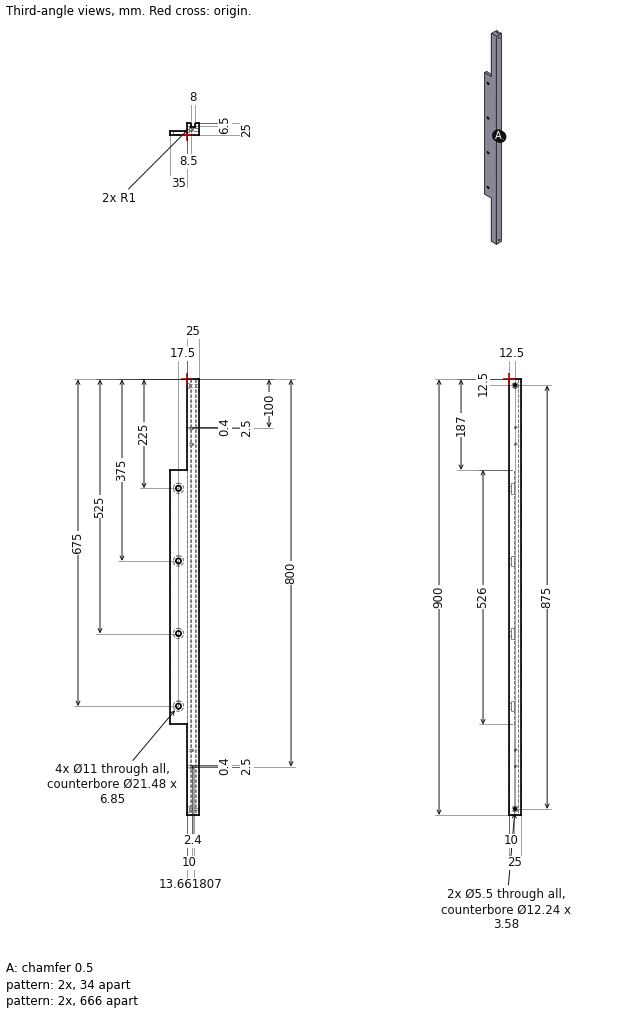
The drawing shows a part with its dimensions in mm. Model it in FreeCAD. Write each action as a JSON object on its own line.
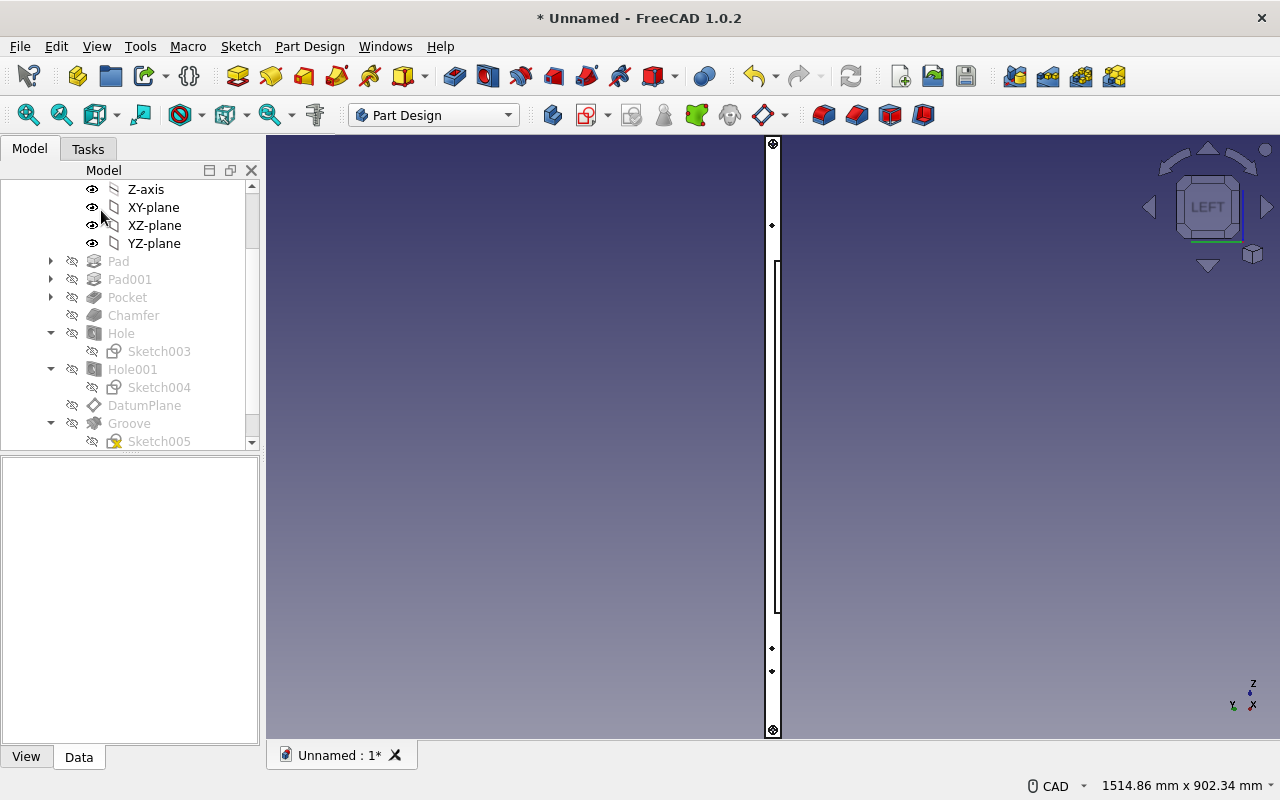
{"action": "scroll", "coordinate": [161, 311], "scroll_direction": "down", "scroll_amount": 3}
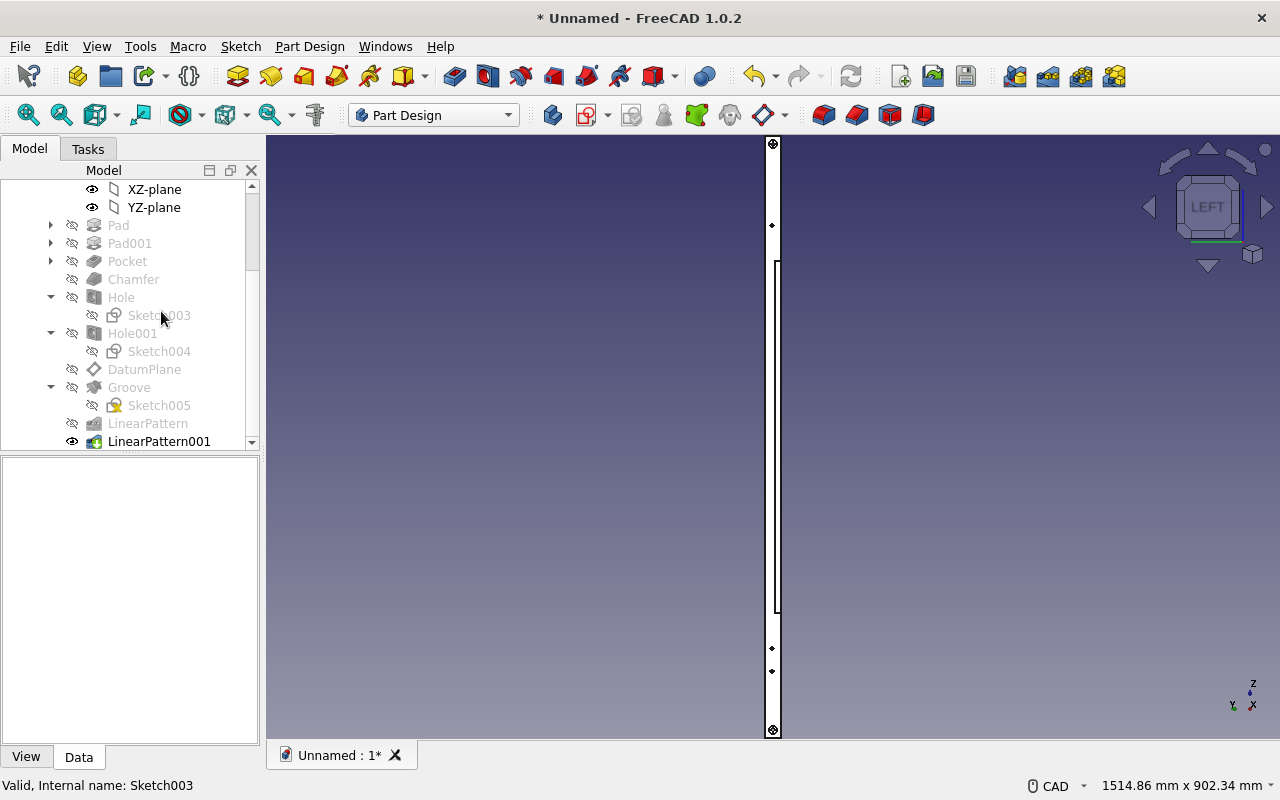
{"action": "scroll", "coordinate": [161, 311], "scroll_direction": "up", "scroll_amount": 15}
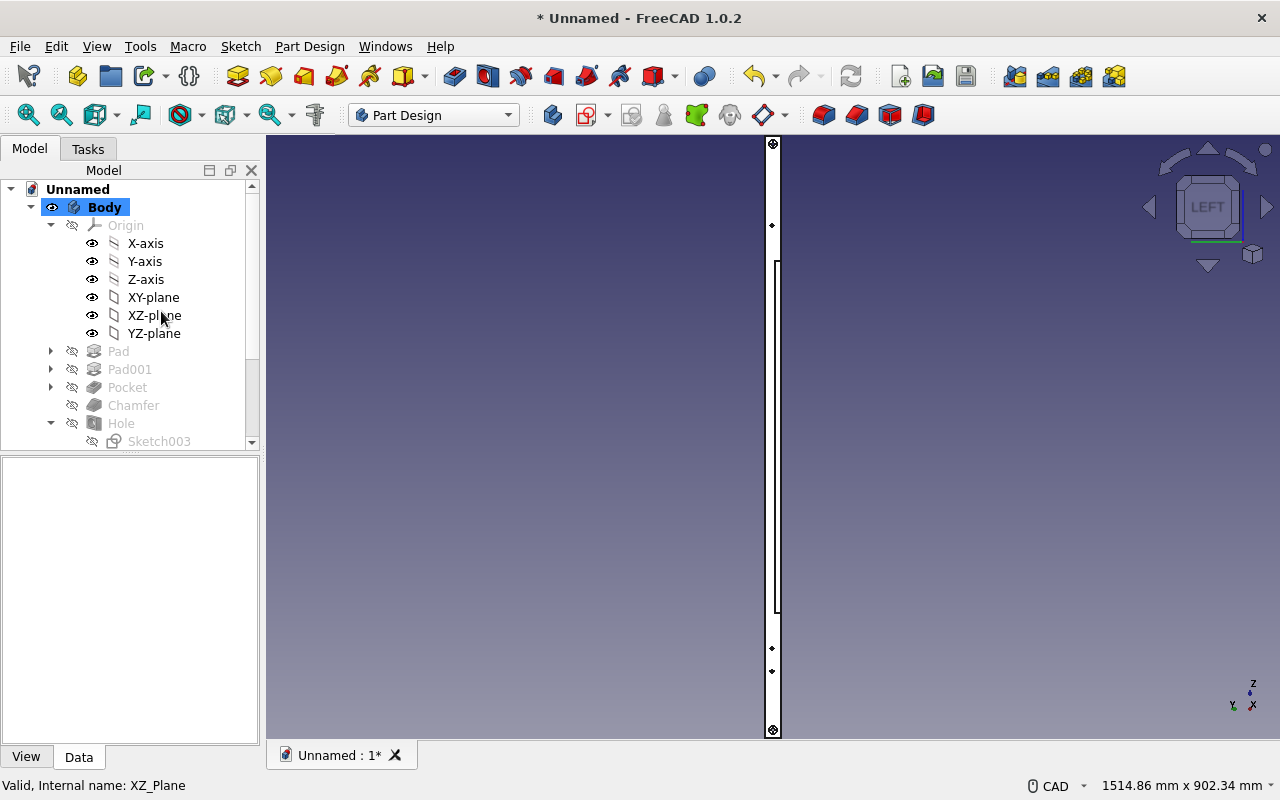
{"action": "left_click", "coordinate": [137, 315]}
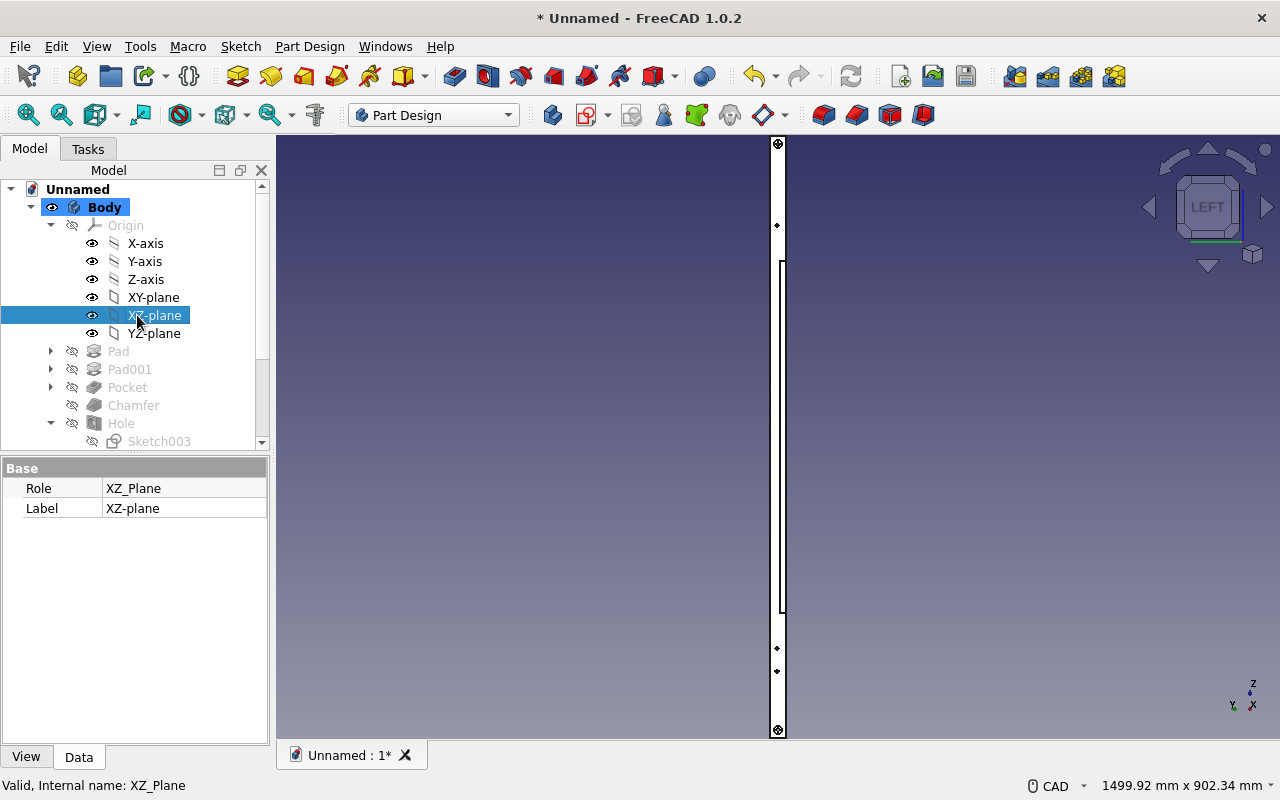
{"action": "left_click", "coordinate": [762, 116]}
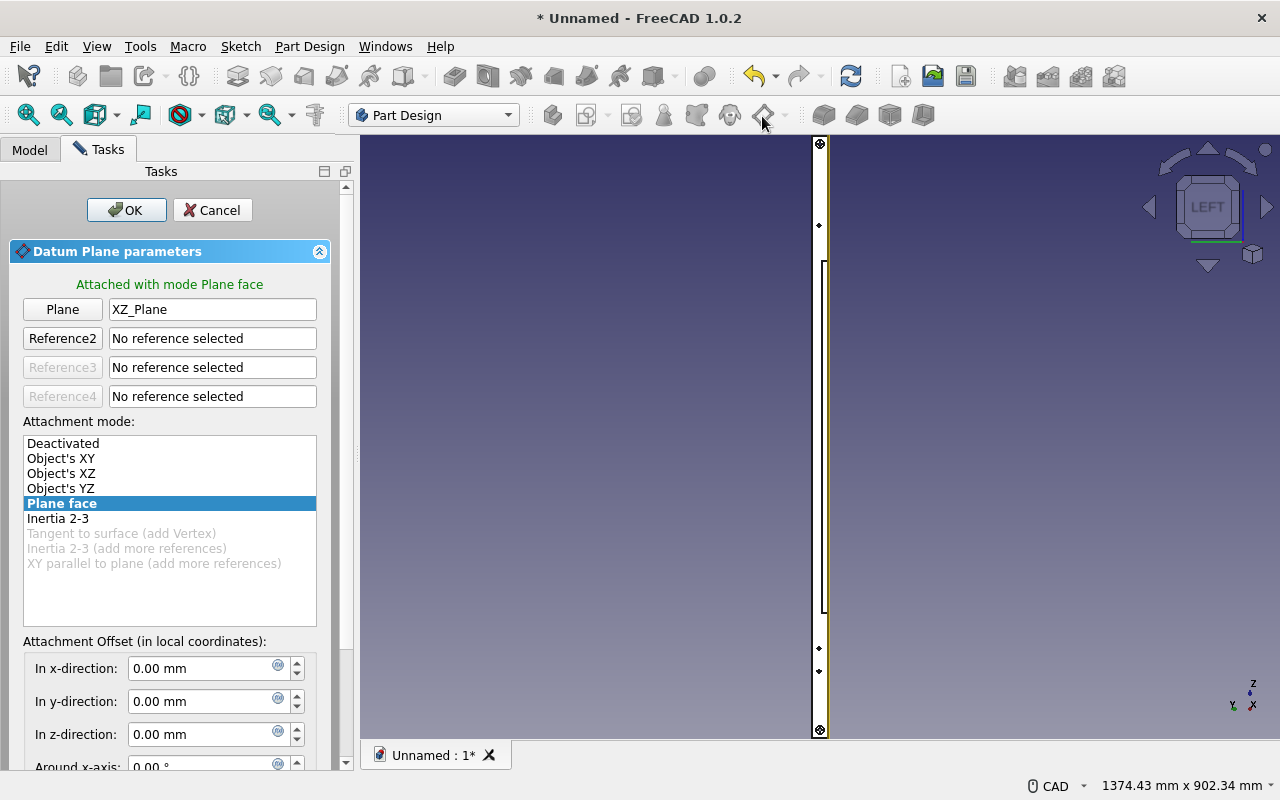
{"action": "triple_click", "coordinate": [210, 734]}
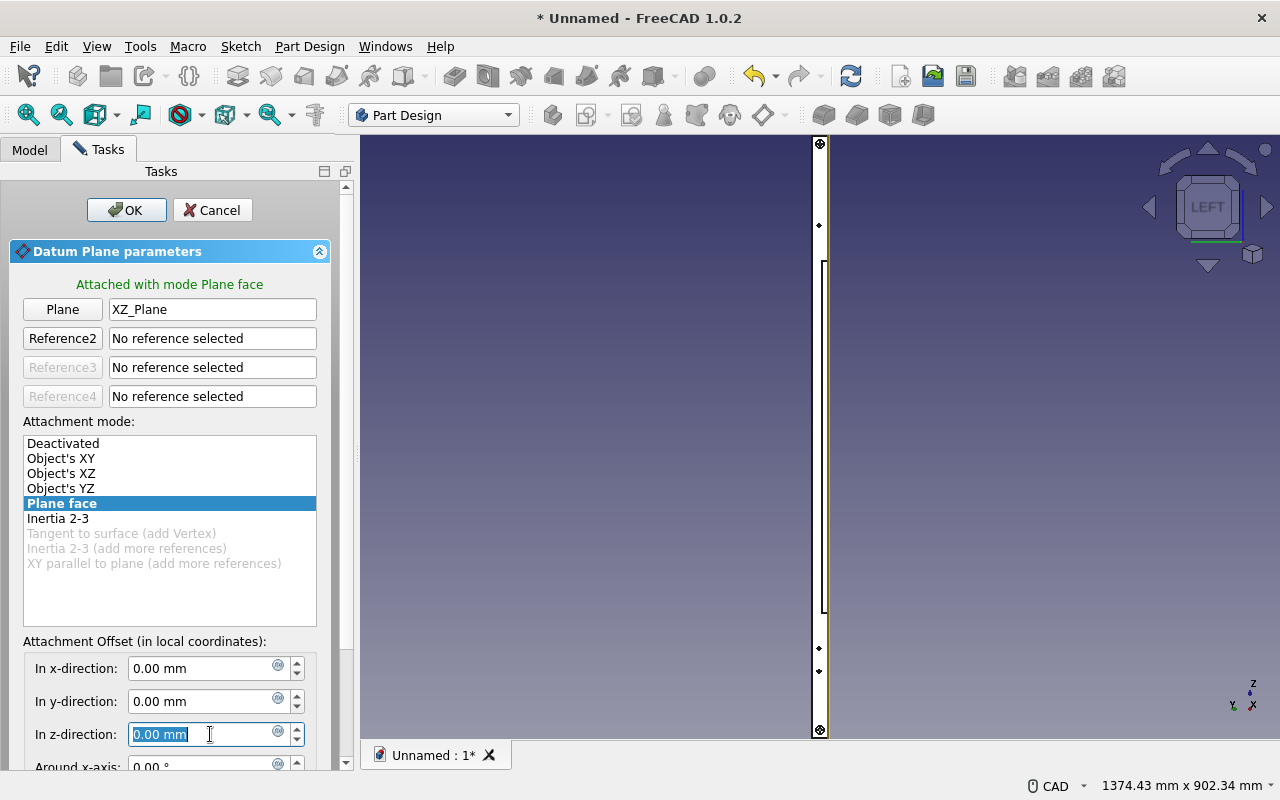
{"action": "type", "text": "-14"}
{"action": "key", "text": "Tab"}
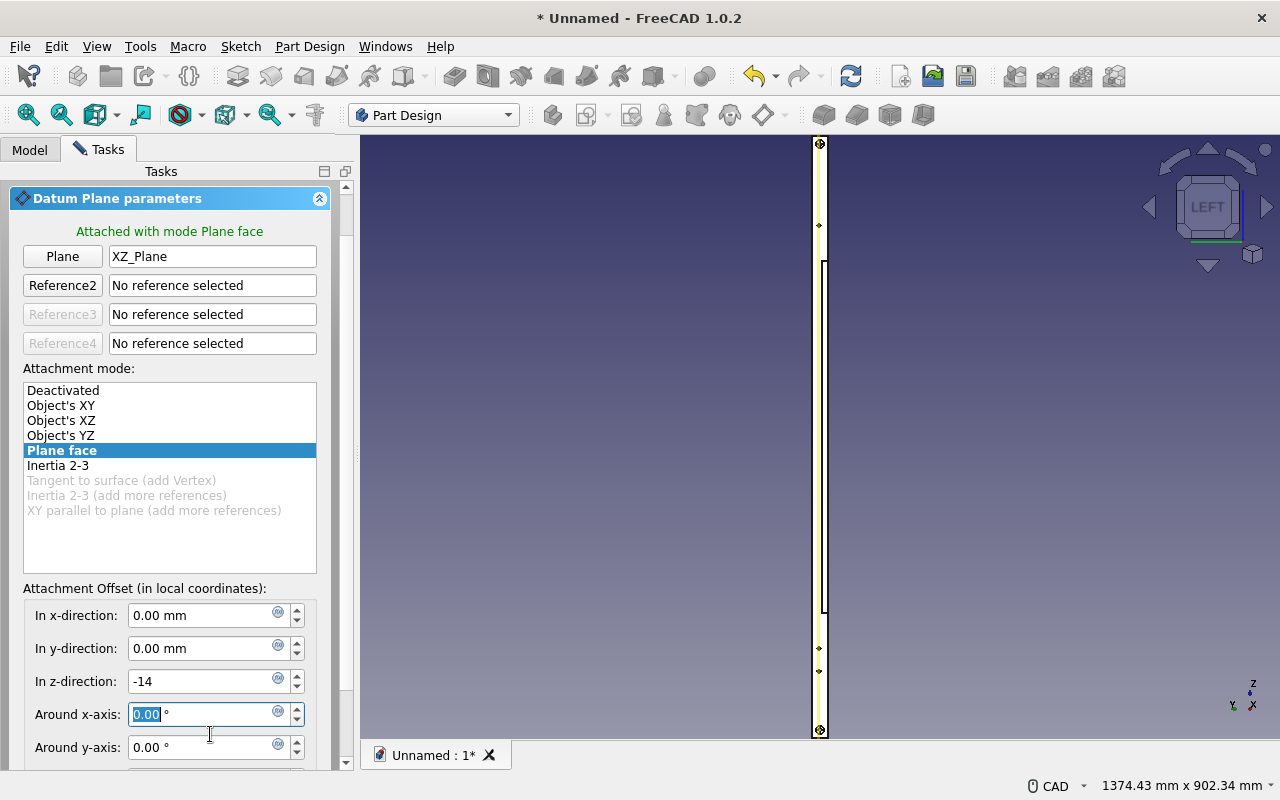
{"action": "scroll", "coordinate": [346, 476], "scroll_direction": "up", "scroll_amount": 2}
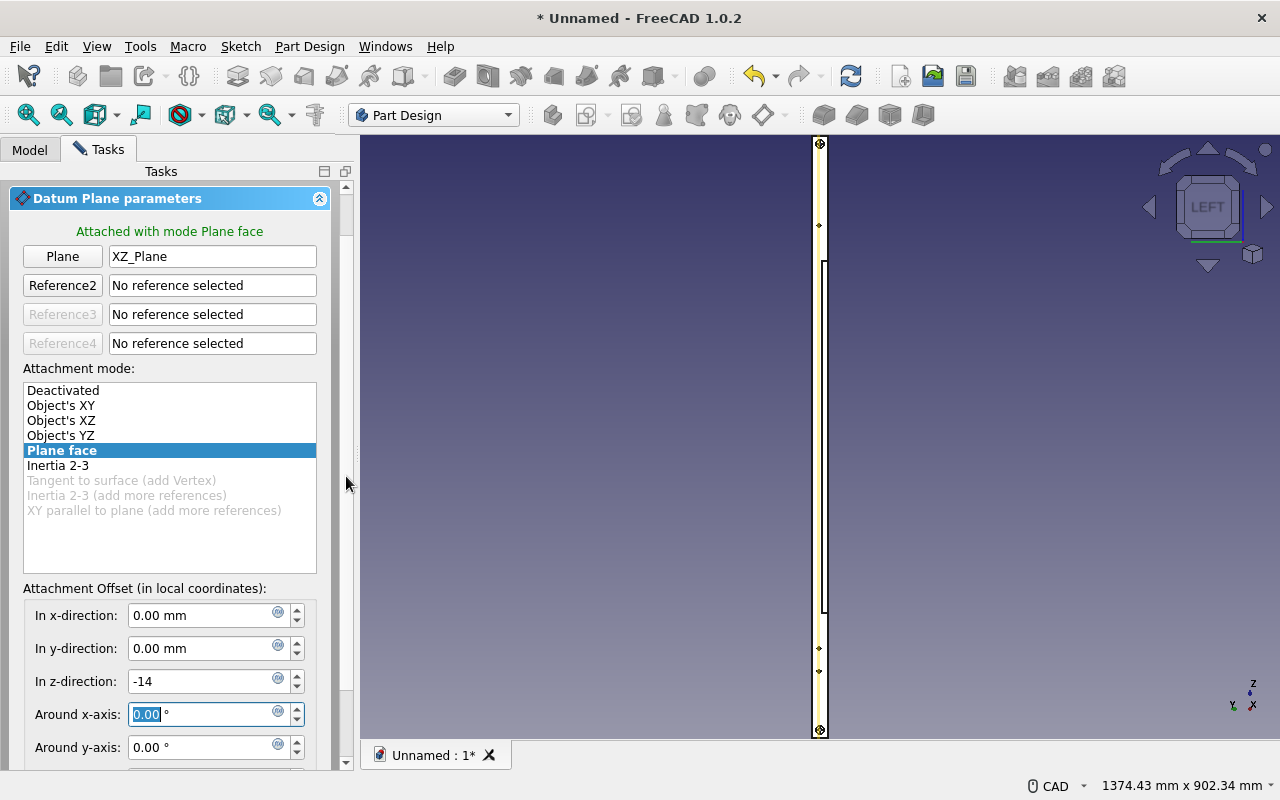
{"action": "left_click", "coordinate": [127, 210]}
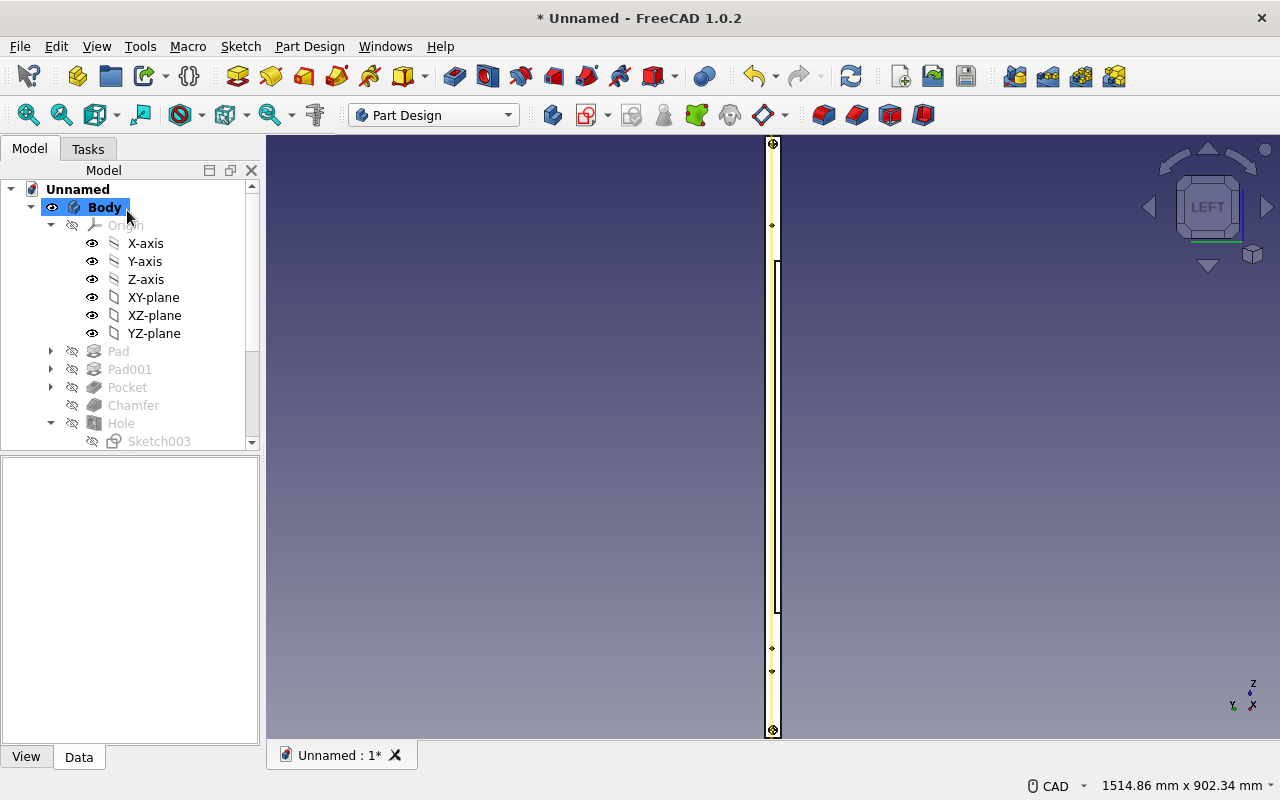
{"action": "scroll", "coordinate": [101, 311], "scroll_direction": "down", "scroll_amount": 3}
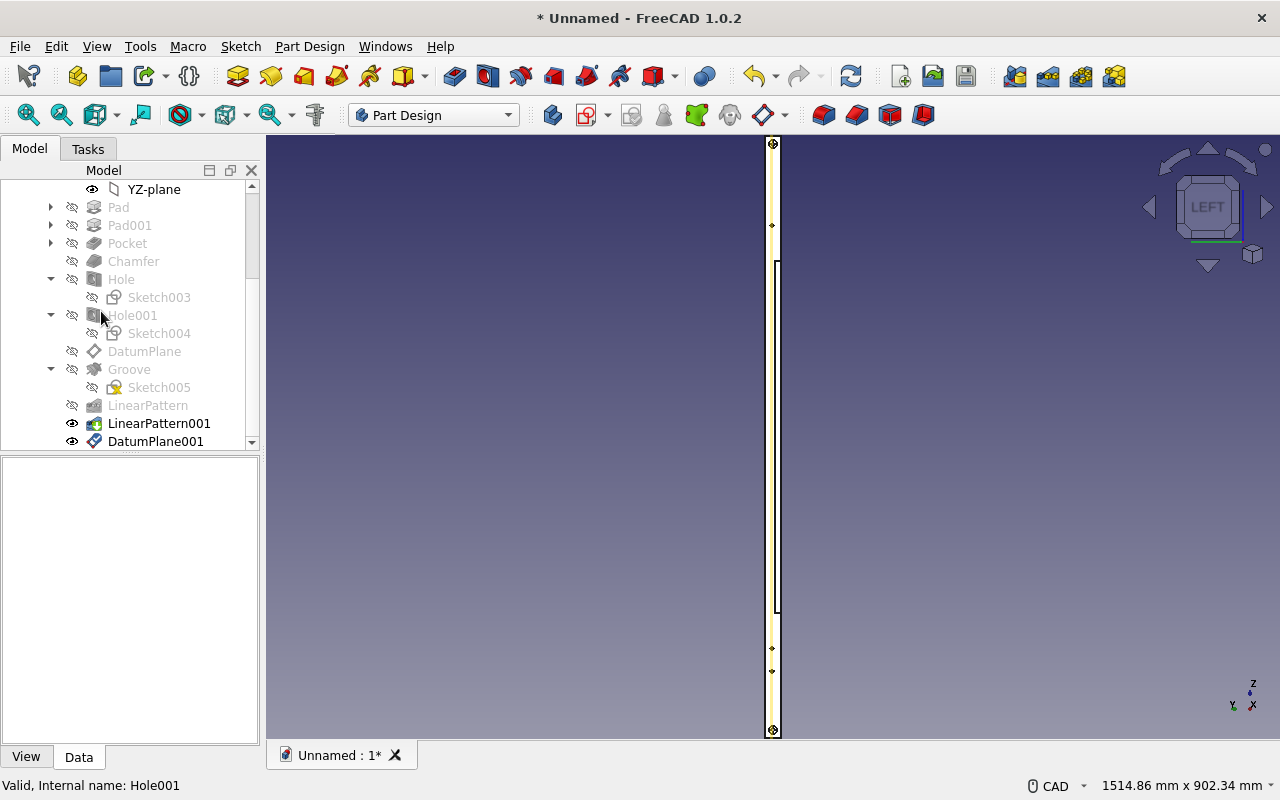
{"action": "left_click", "coordinate": [117, 441]}